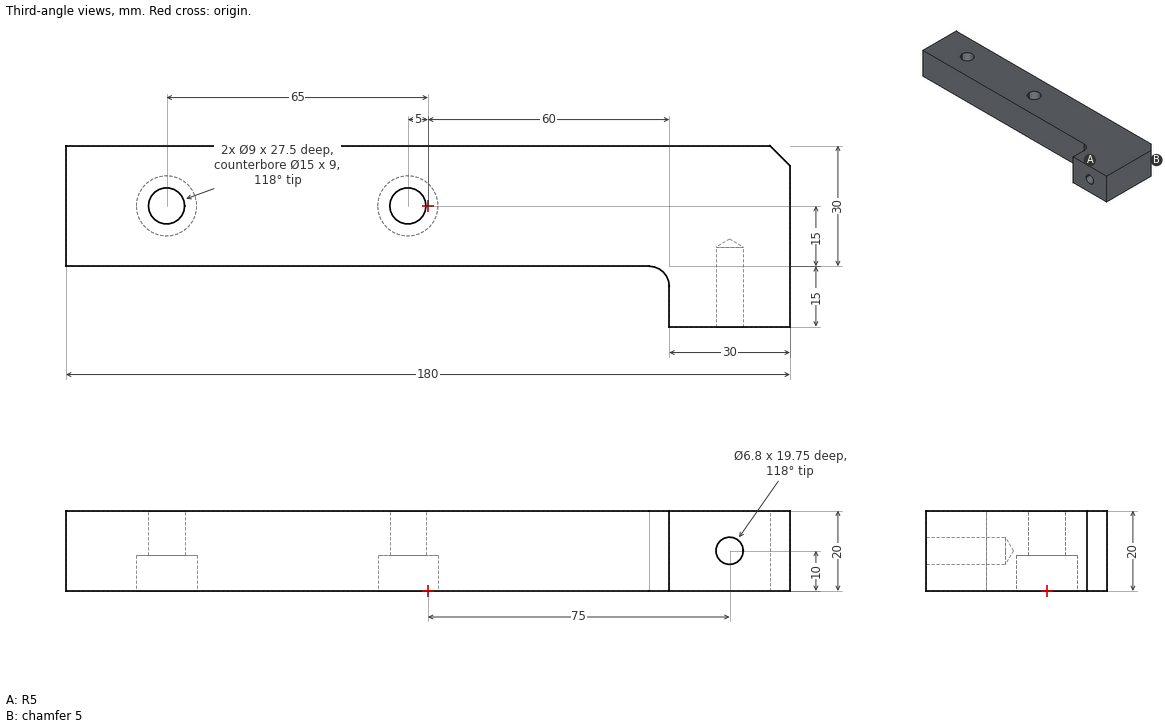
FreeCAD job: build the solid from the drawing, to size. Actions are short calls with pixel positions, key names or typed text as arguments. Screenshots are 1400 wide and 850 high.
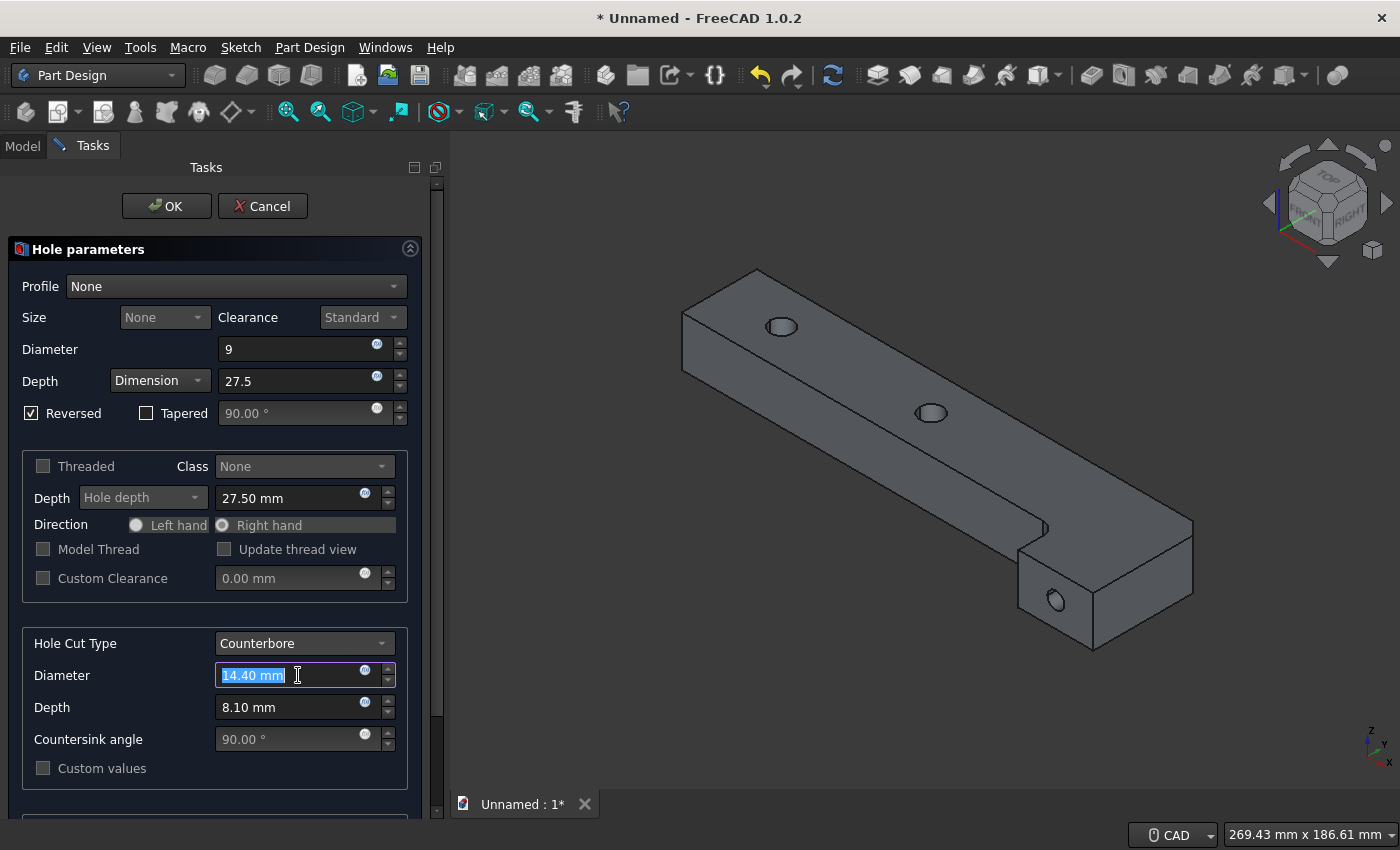
text(15)
key(Tab)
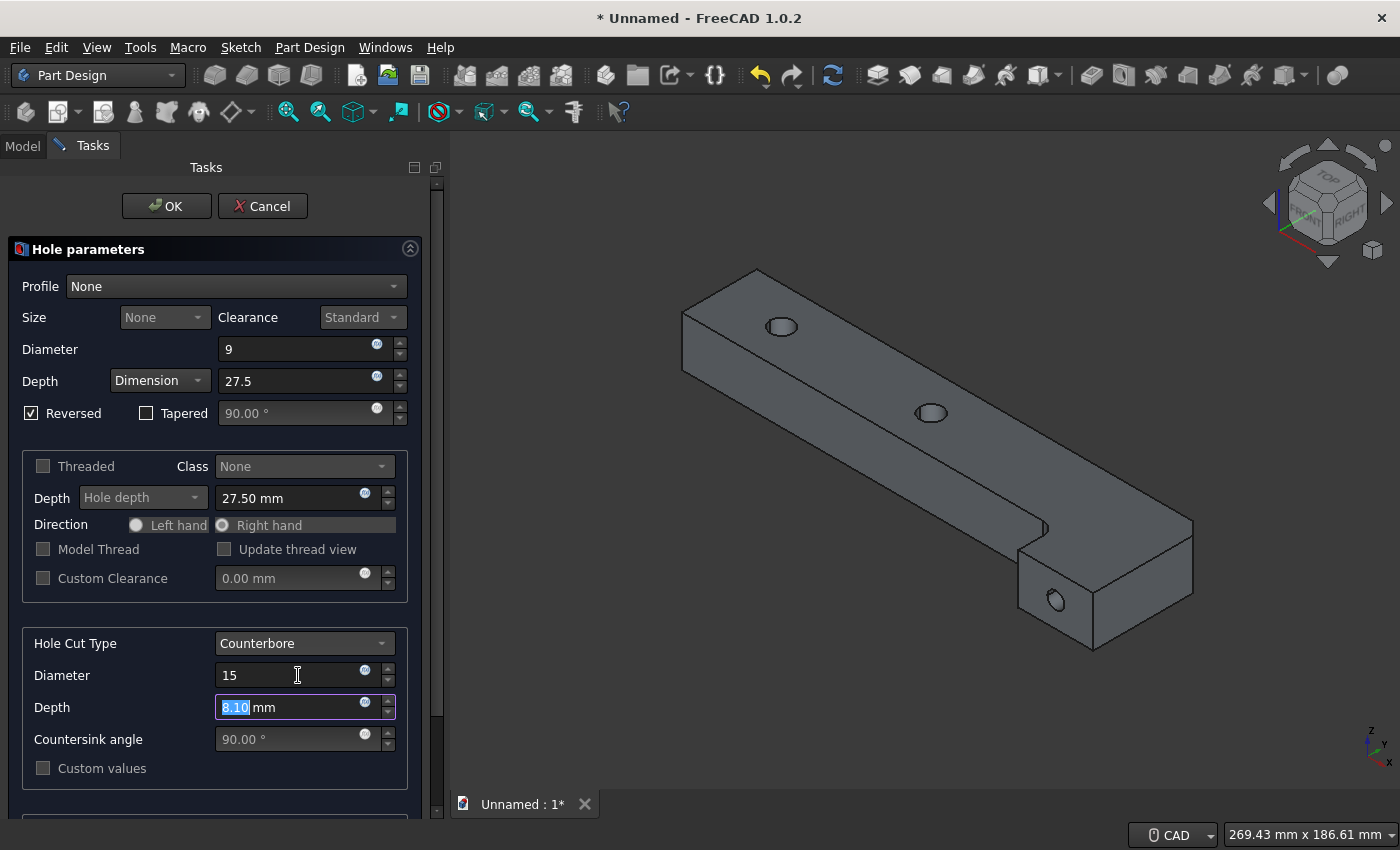
text(9)
key(Tab)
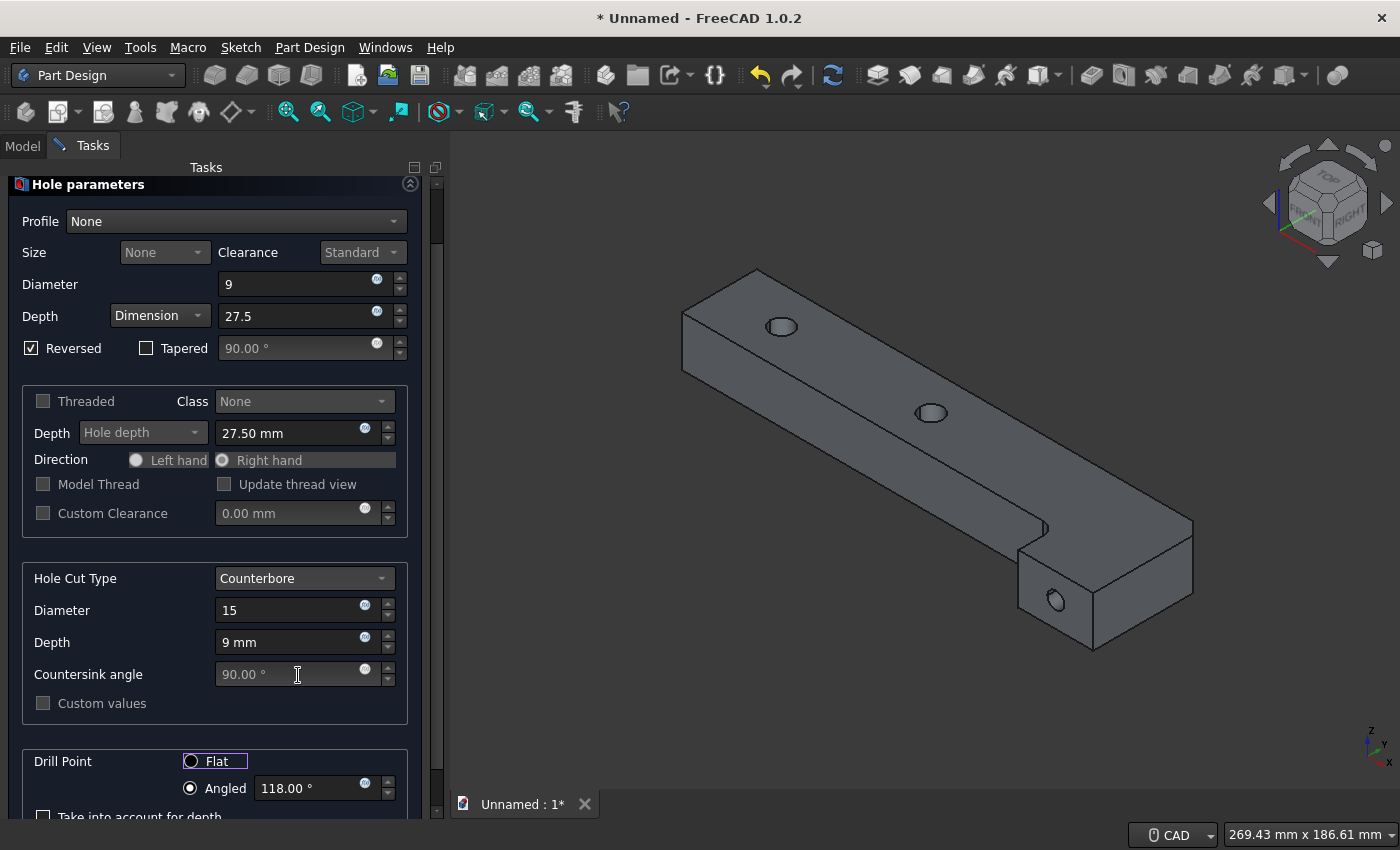
scroll(437, 498, up, 2)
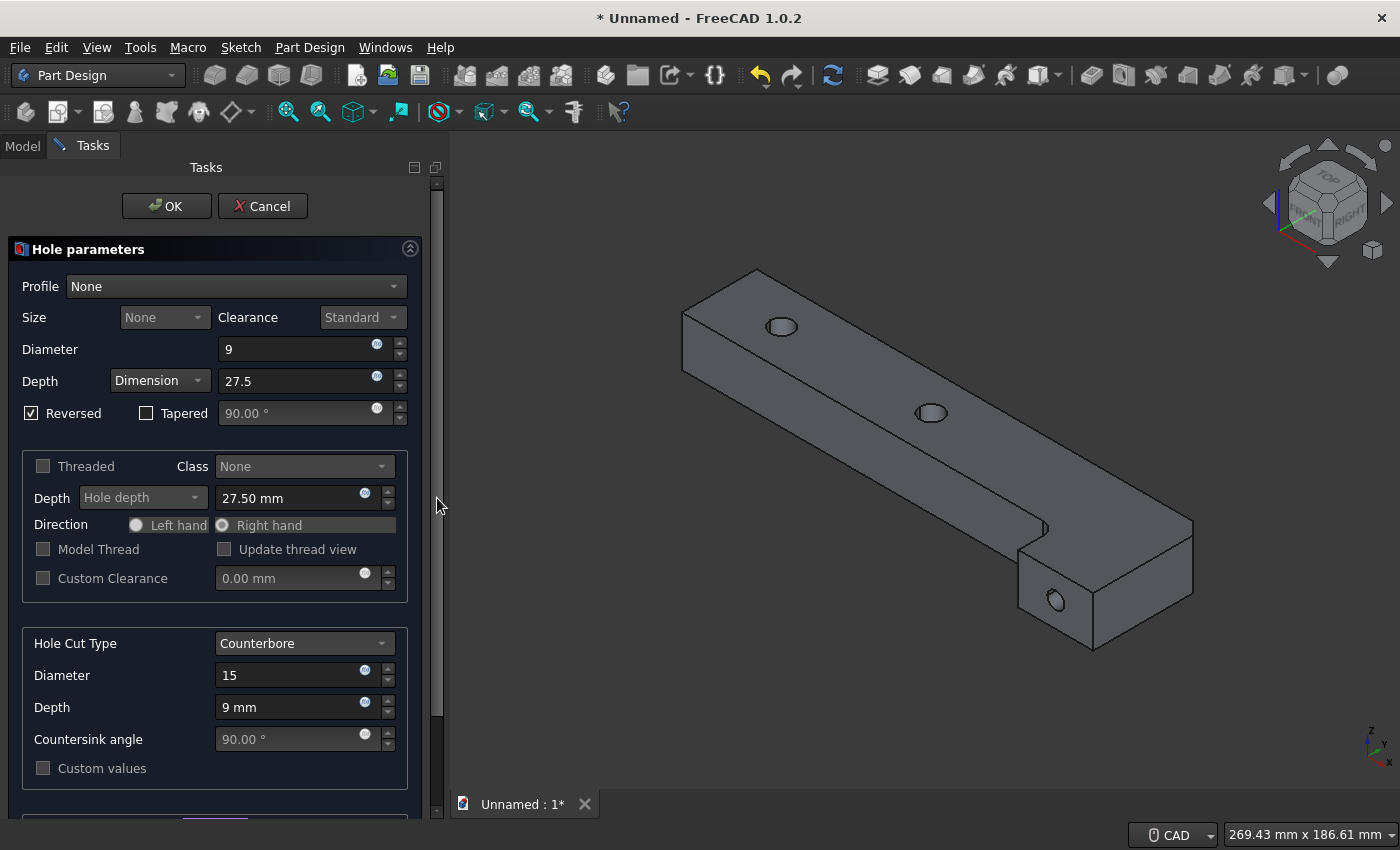
click(167, 206)